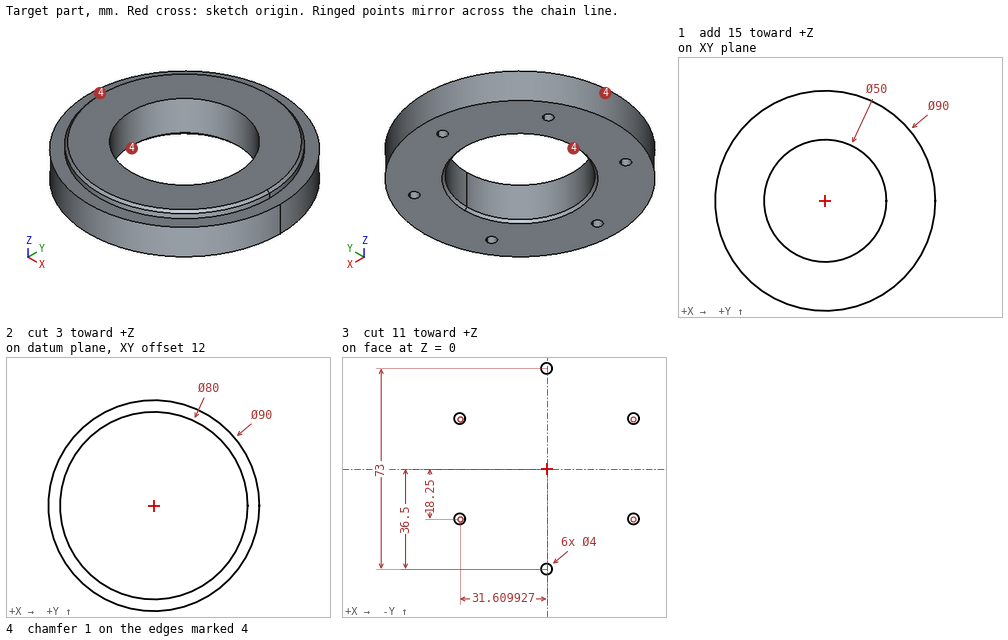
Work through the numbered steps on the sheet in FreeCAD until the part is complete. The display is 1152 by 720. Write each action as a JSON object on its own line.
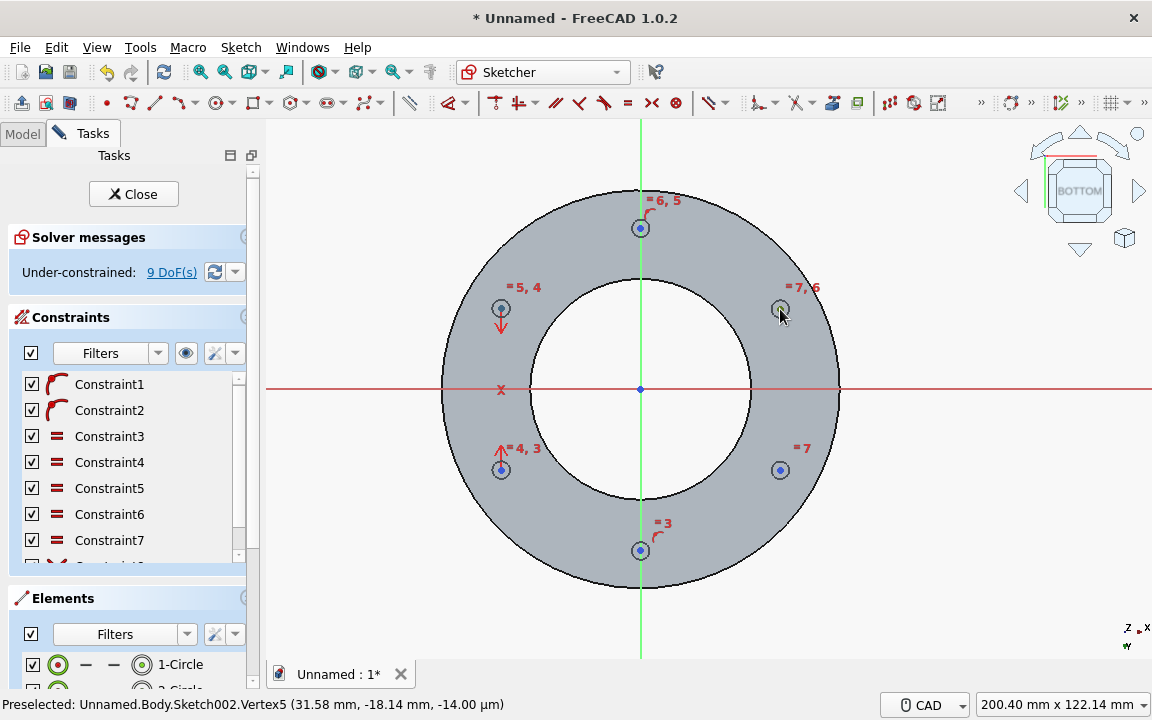
{"action": "left_click", "coordinate": [641, 596]}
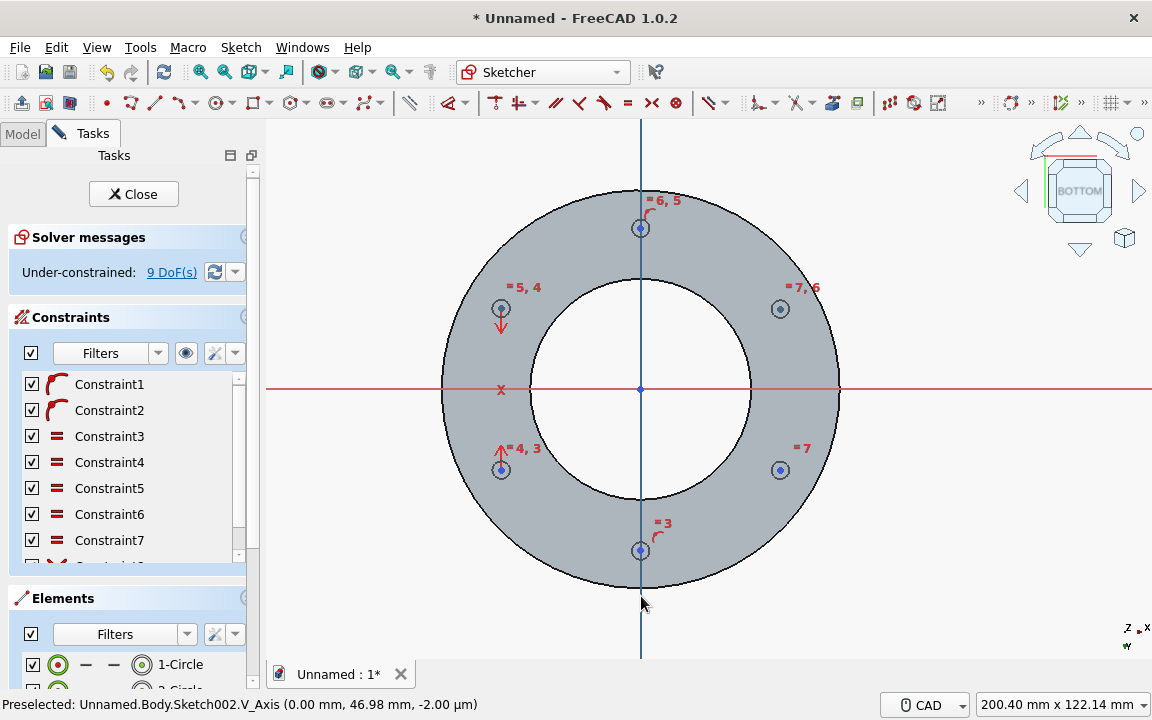
{"action": "left_click", "coordinate": [652, 104]}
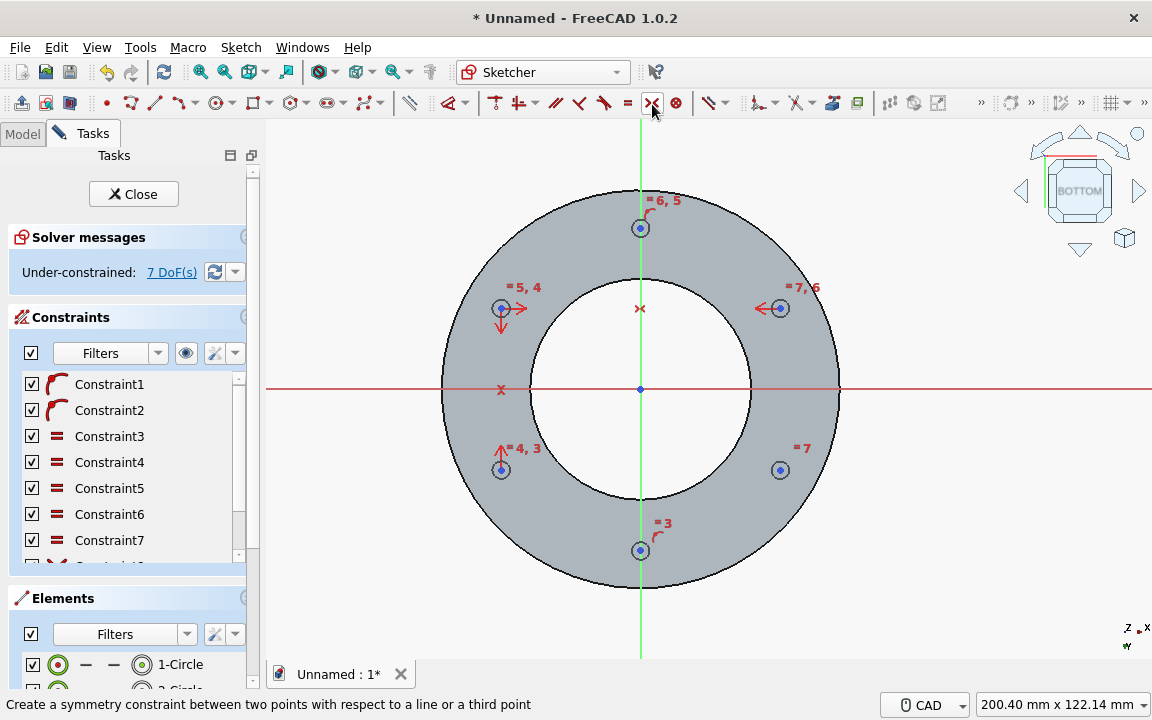
{"action": "left_click", "coordinate": [501, 470]}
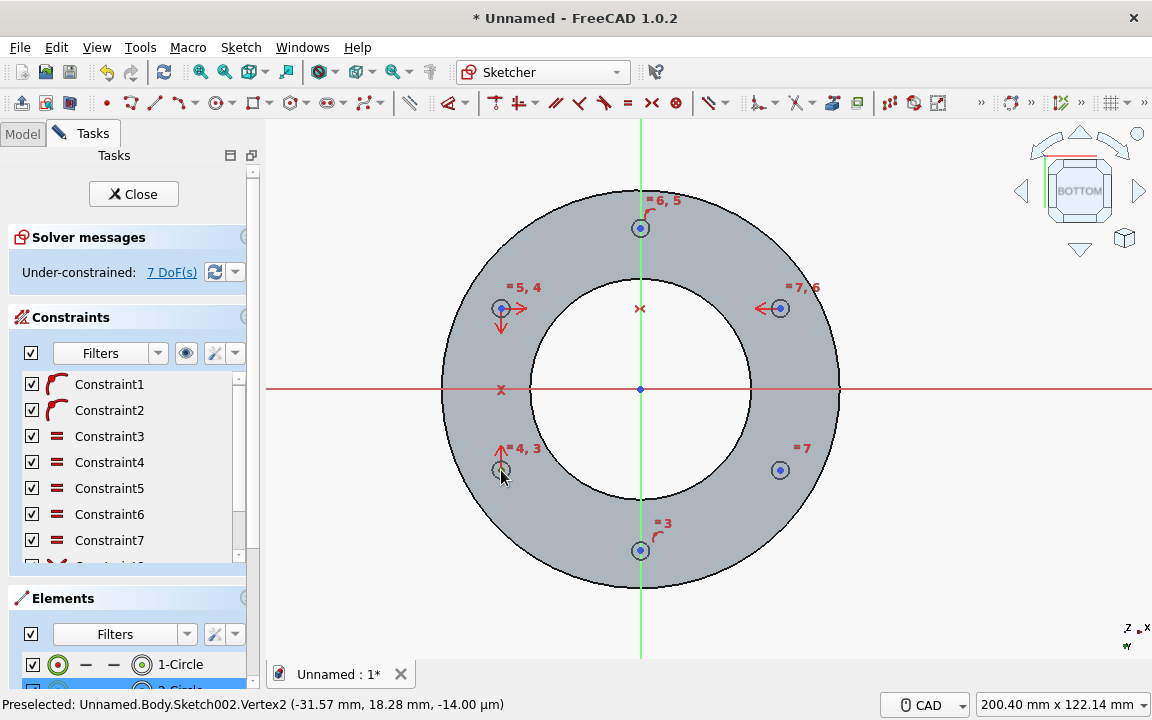
{"action": "left_click", "coordinate": [780, 470]}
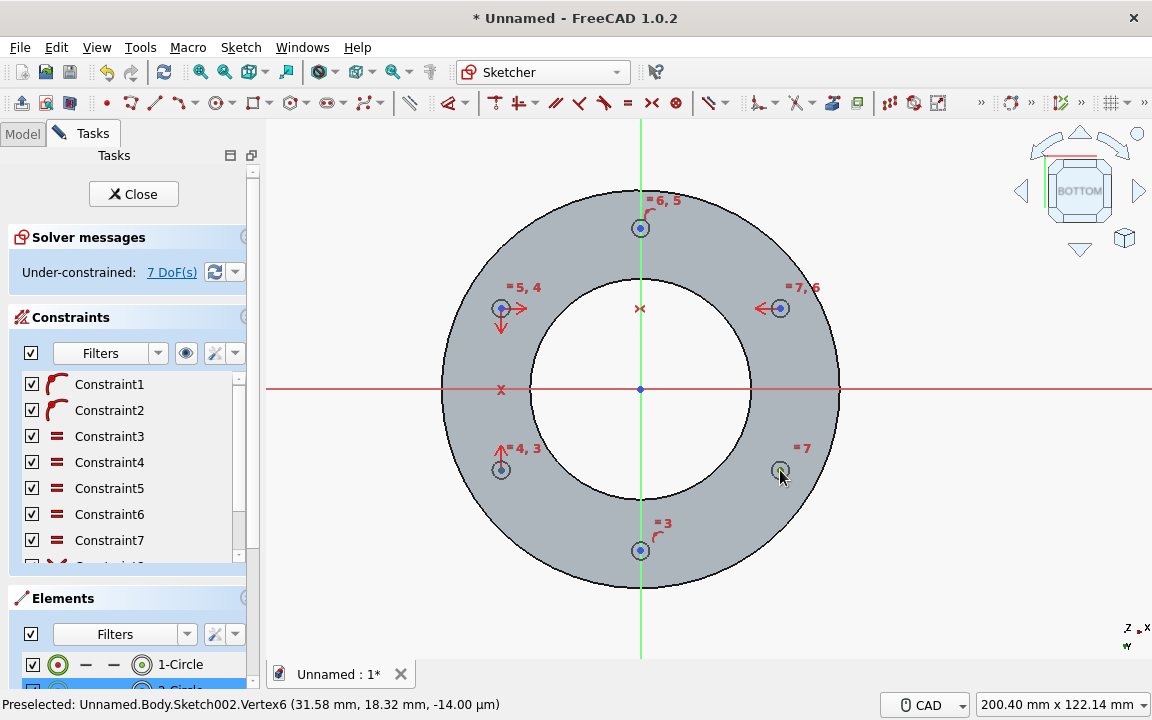
{"action": "left_click", "coordinate": [641, 596]}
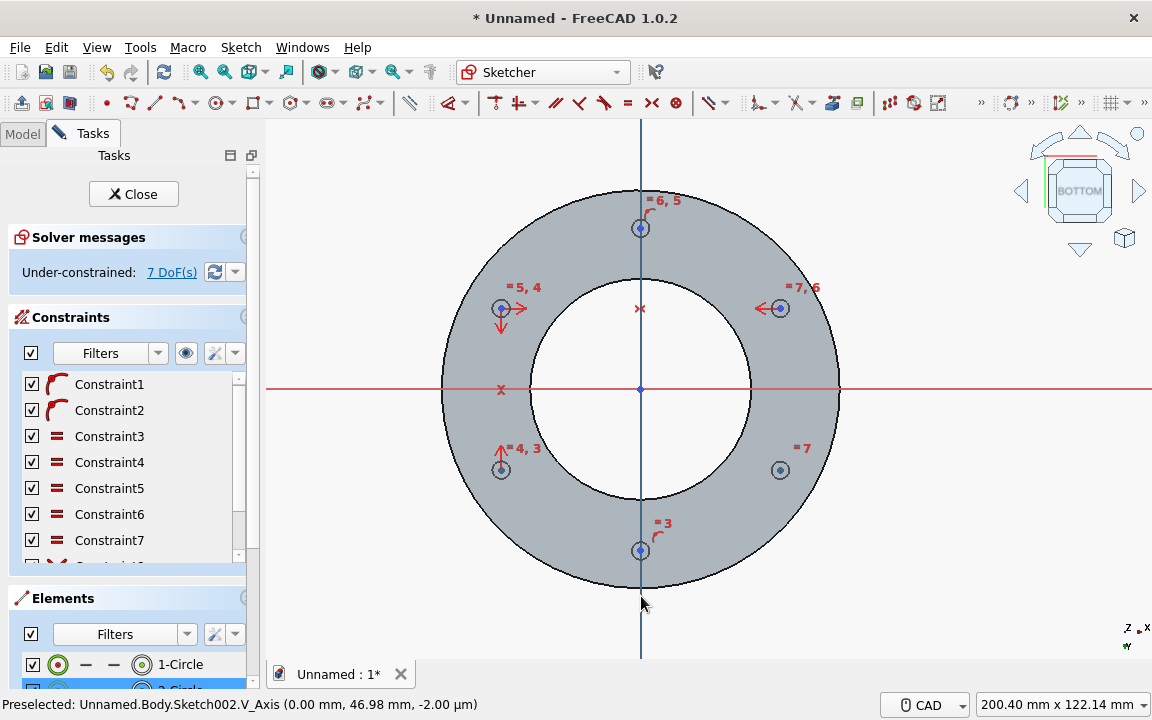
{"action": "left_click", "coordinate": [652, 104]}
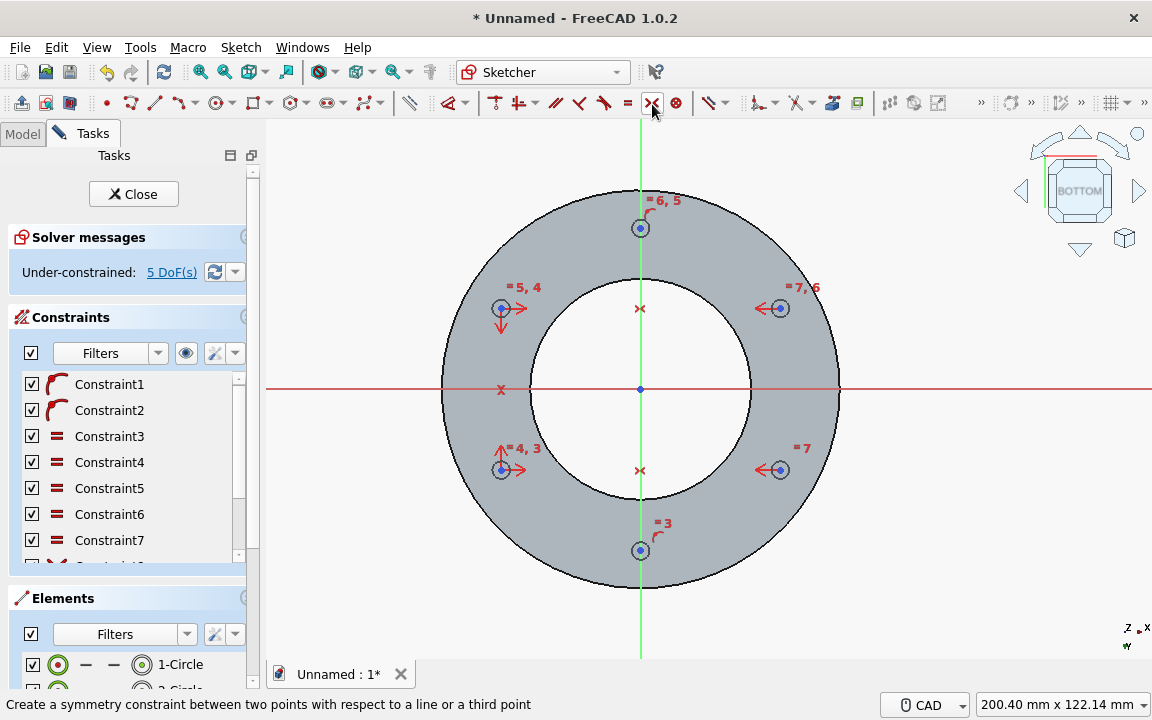
{"action": "left_click", "coordinate": [448, 104]}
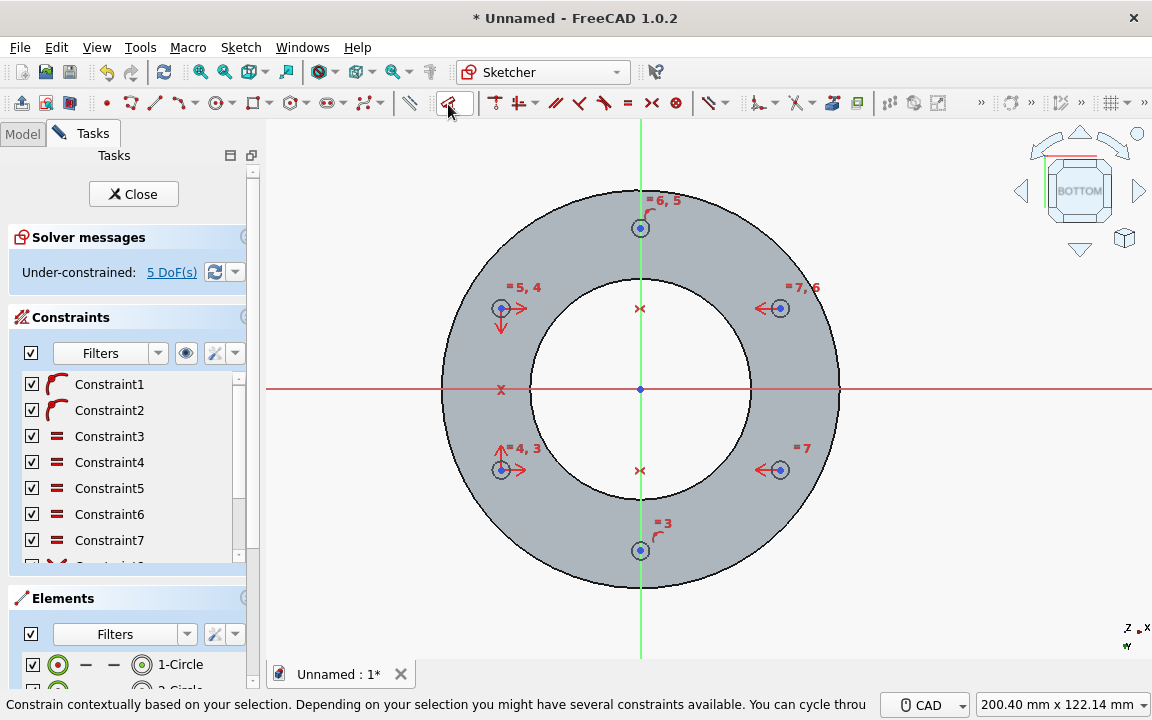
{"action": "scroll", "coordinate": [641, 542], "scroll_direction": "up", "scroll_amount": 5}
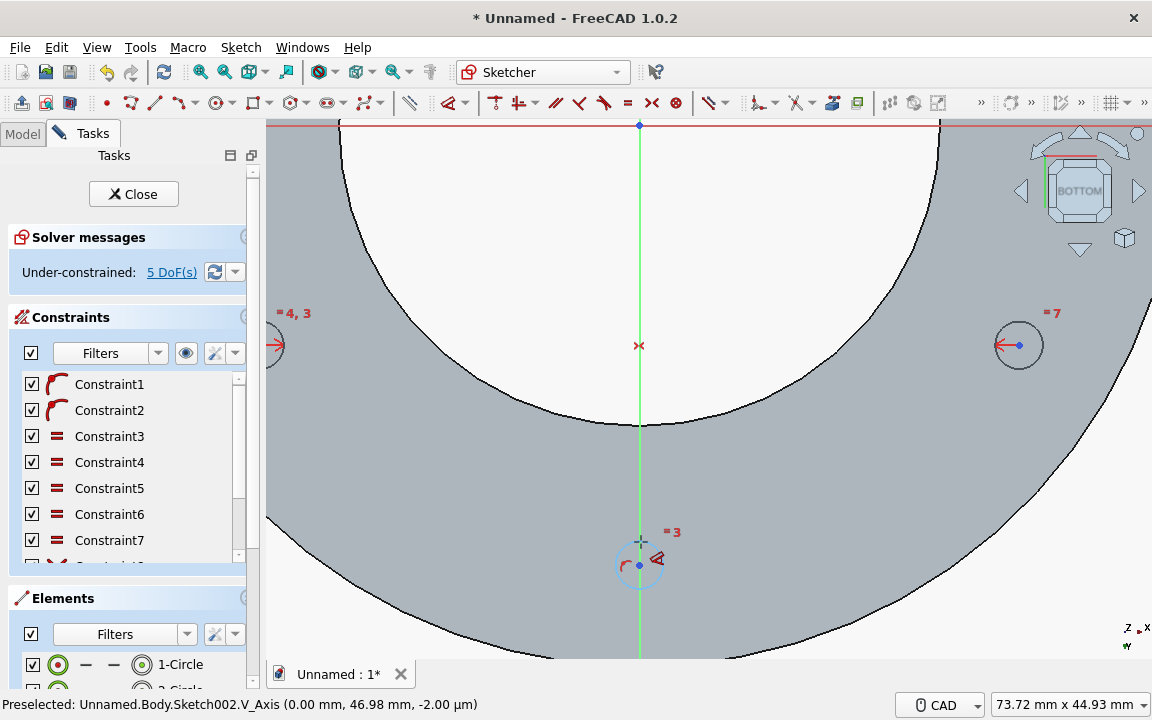
{"action": "left_click", "coordinate": [640, 541]}
{"action": "left_click", "coordinate": [667, 516]}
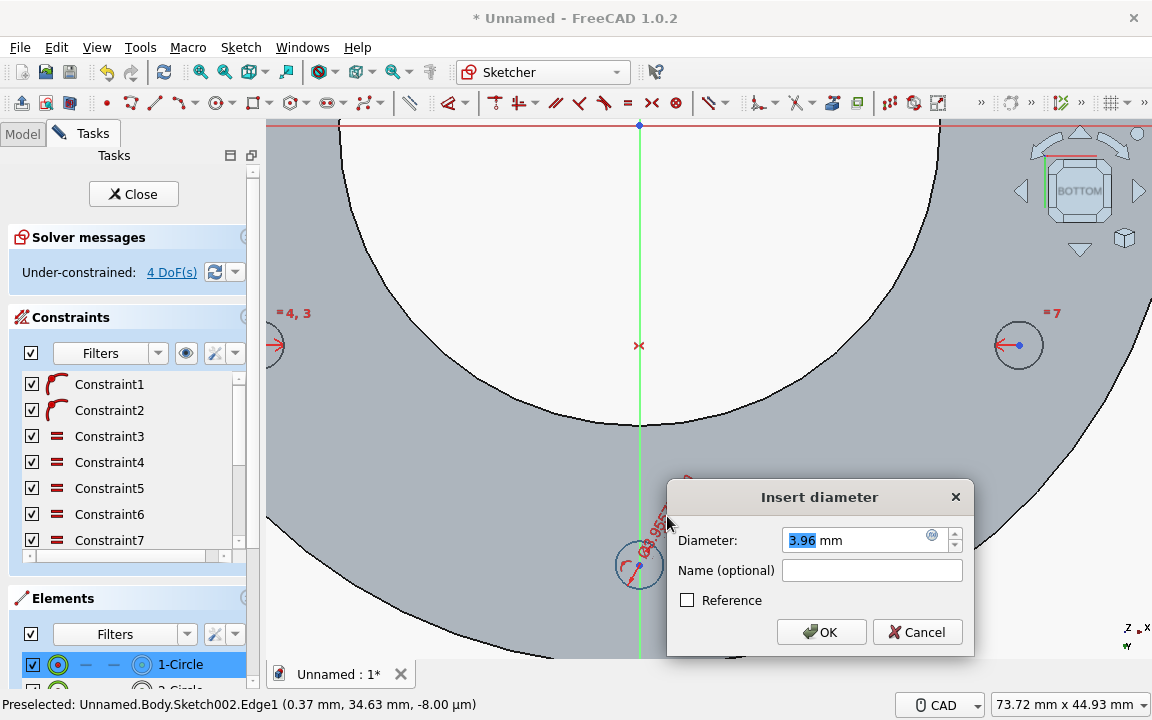
{"action": "type", "text": "4"}
{"action": "key", "text": "Return"}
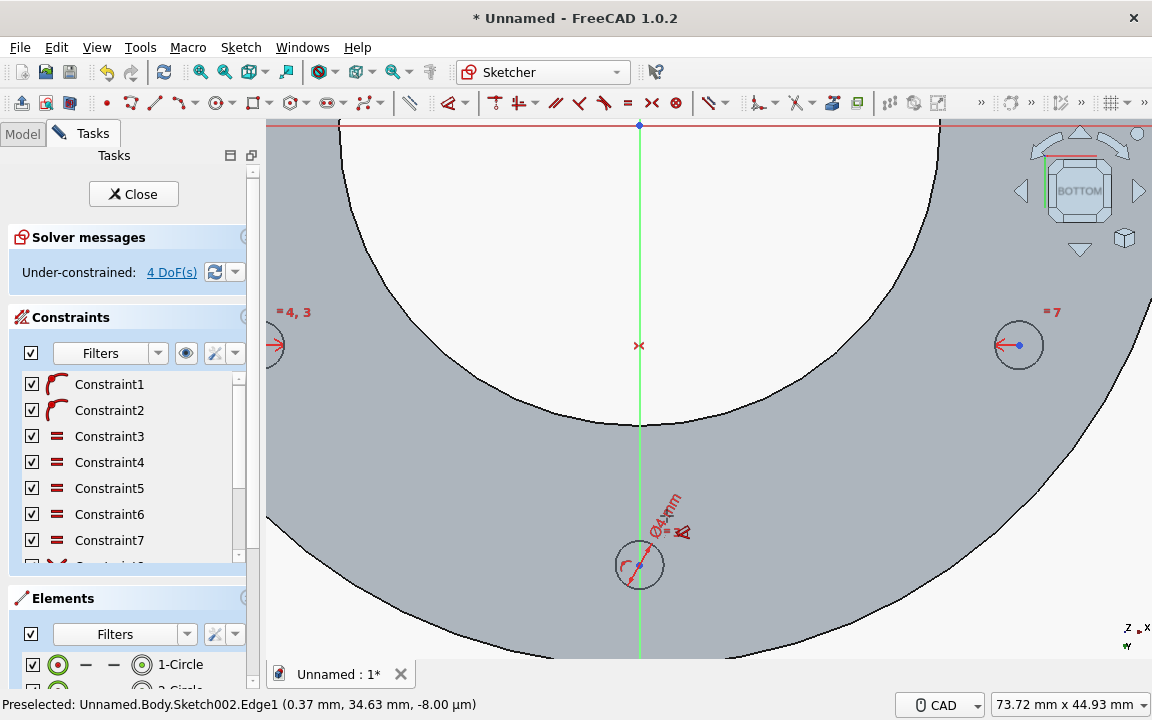
{"action": "left_click", "coordinate": [640, 565]}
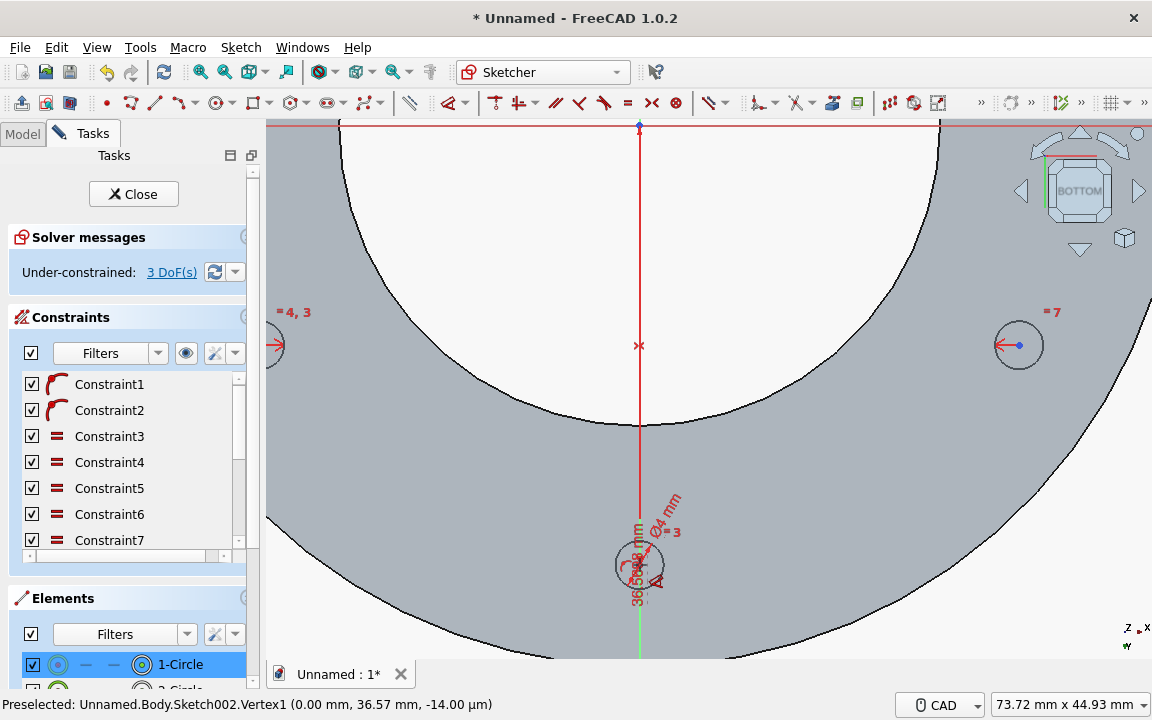
{"action": "scroll", "coordinate": [641, 542], "scroll_direction": "down", "scroll_amount": 5}